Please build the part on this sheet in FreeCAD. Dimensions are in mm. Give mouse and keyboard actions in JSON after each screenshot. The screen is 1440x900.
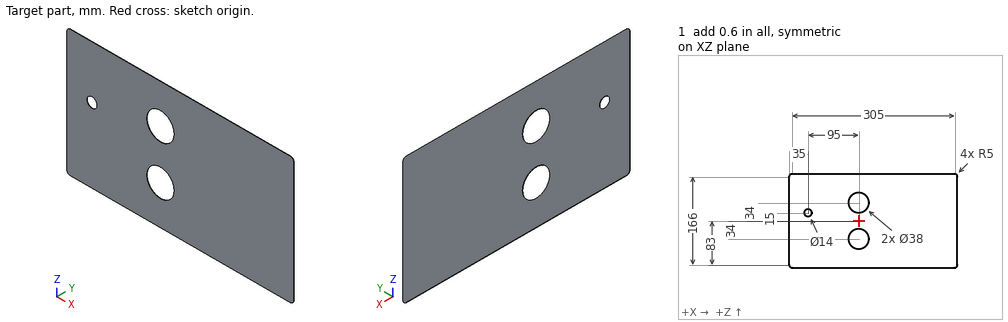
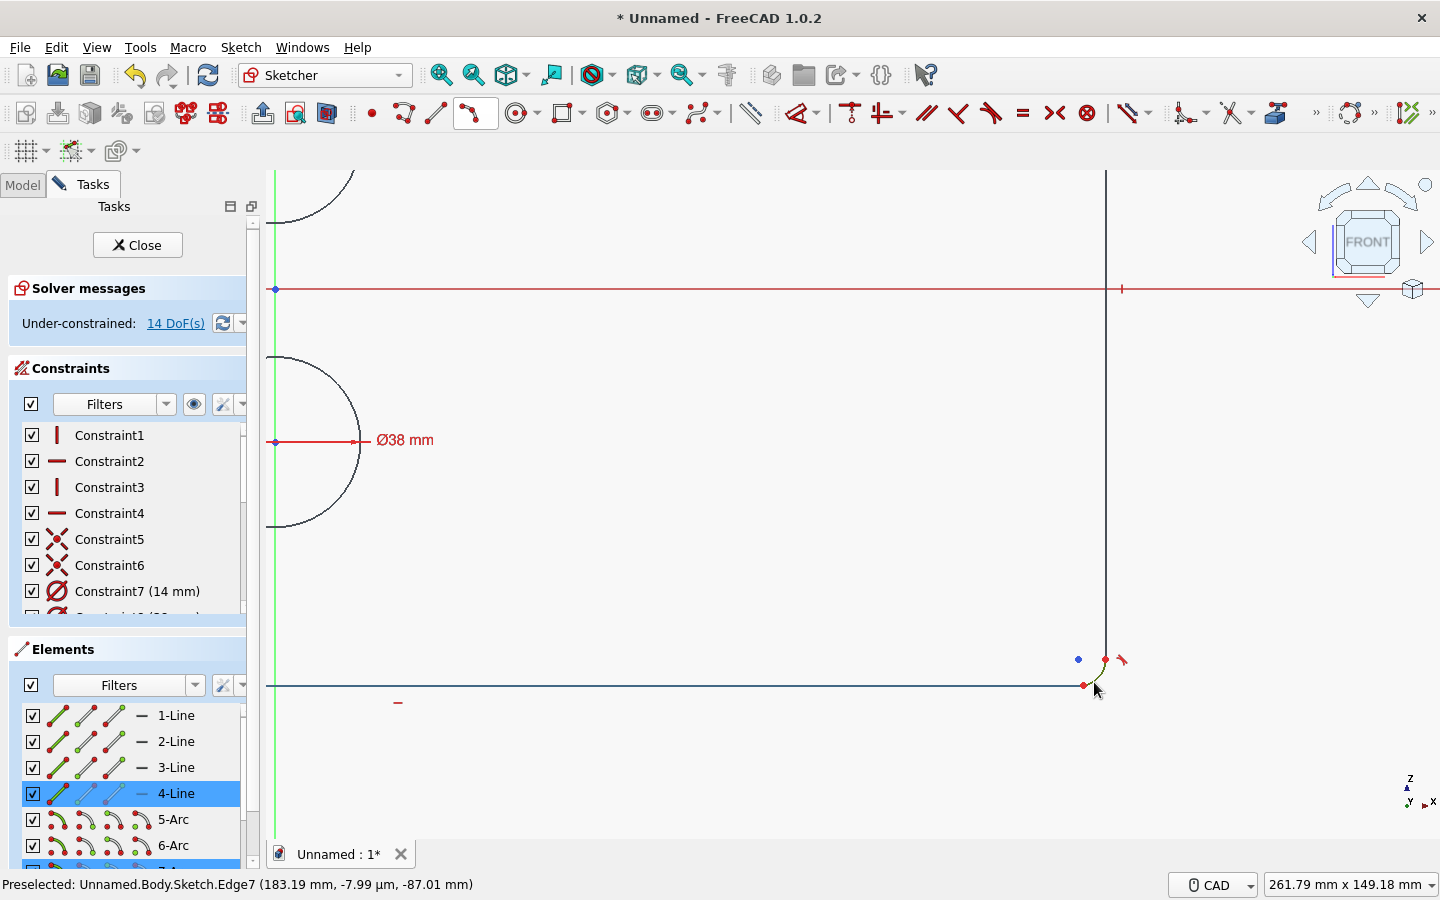
{"action": "left_click", "coordinate": [992, 114]}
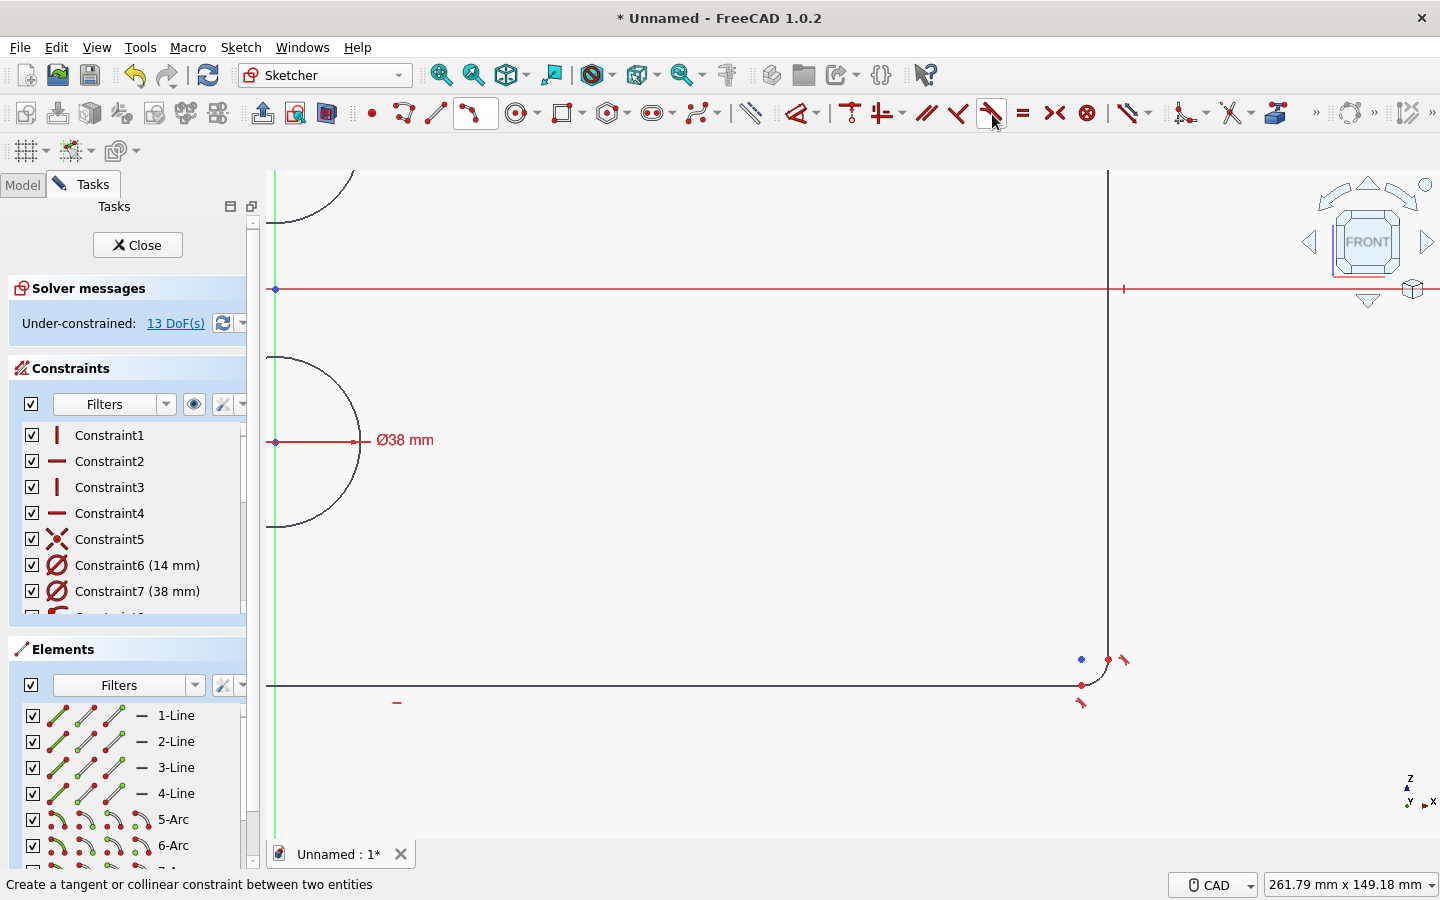
{"action": "left_click", "coordinate": [671, 686]}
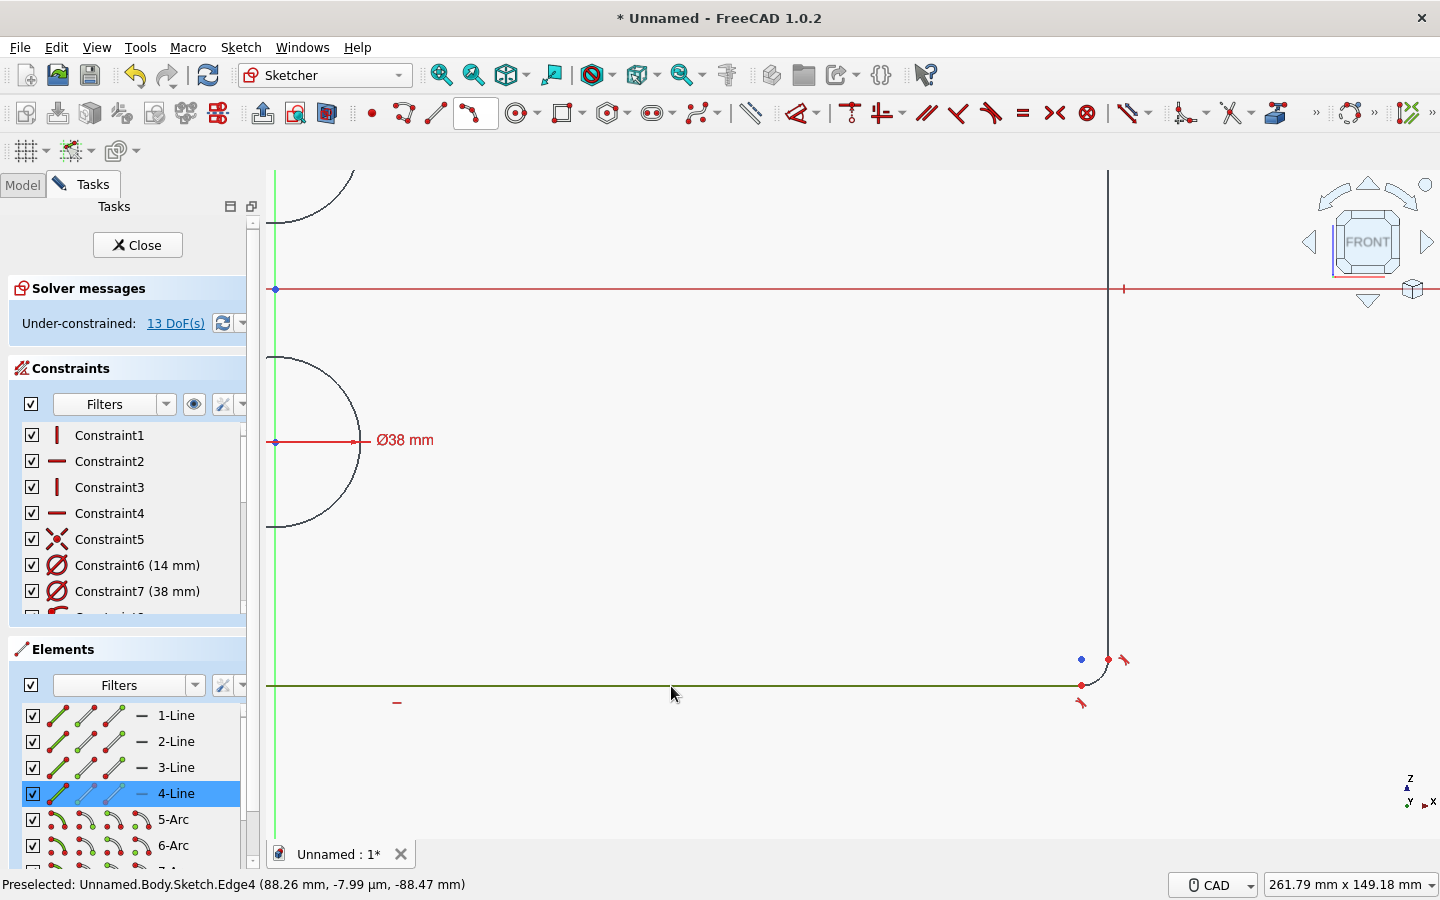
{"action": "scroll", "coordinate": [1099, 680], "scroll_direction": "down", "scroll_amount": 4}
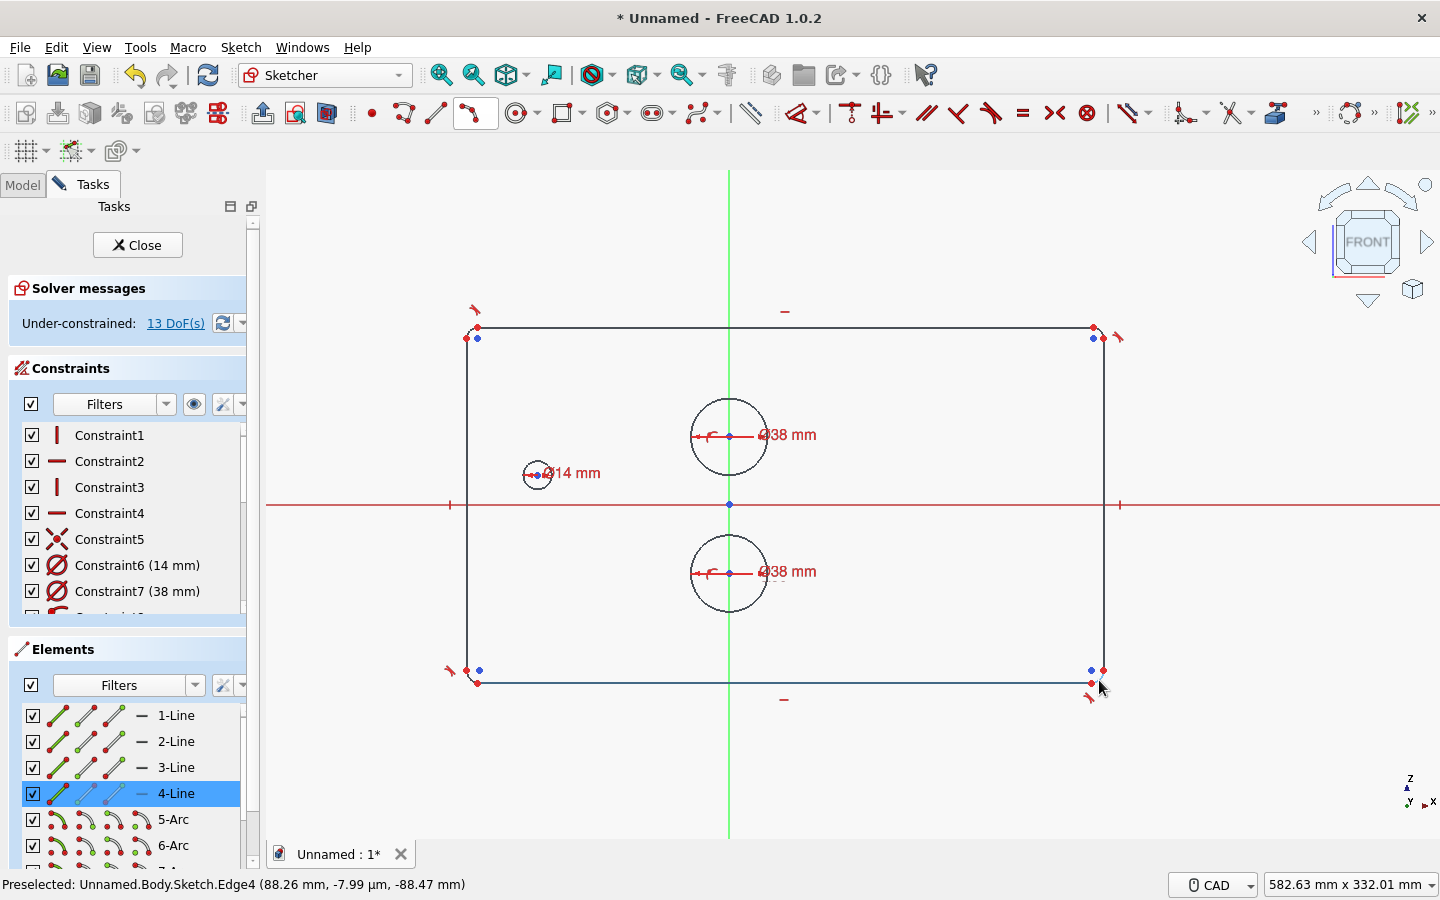
{"action": "scroll", "coordinate": [468, 676], "scroll_direction": "up", "scroll_amount": 5}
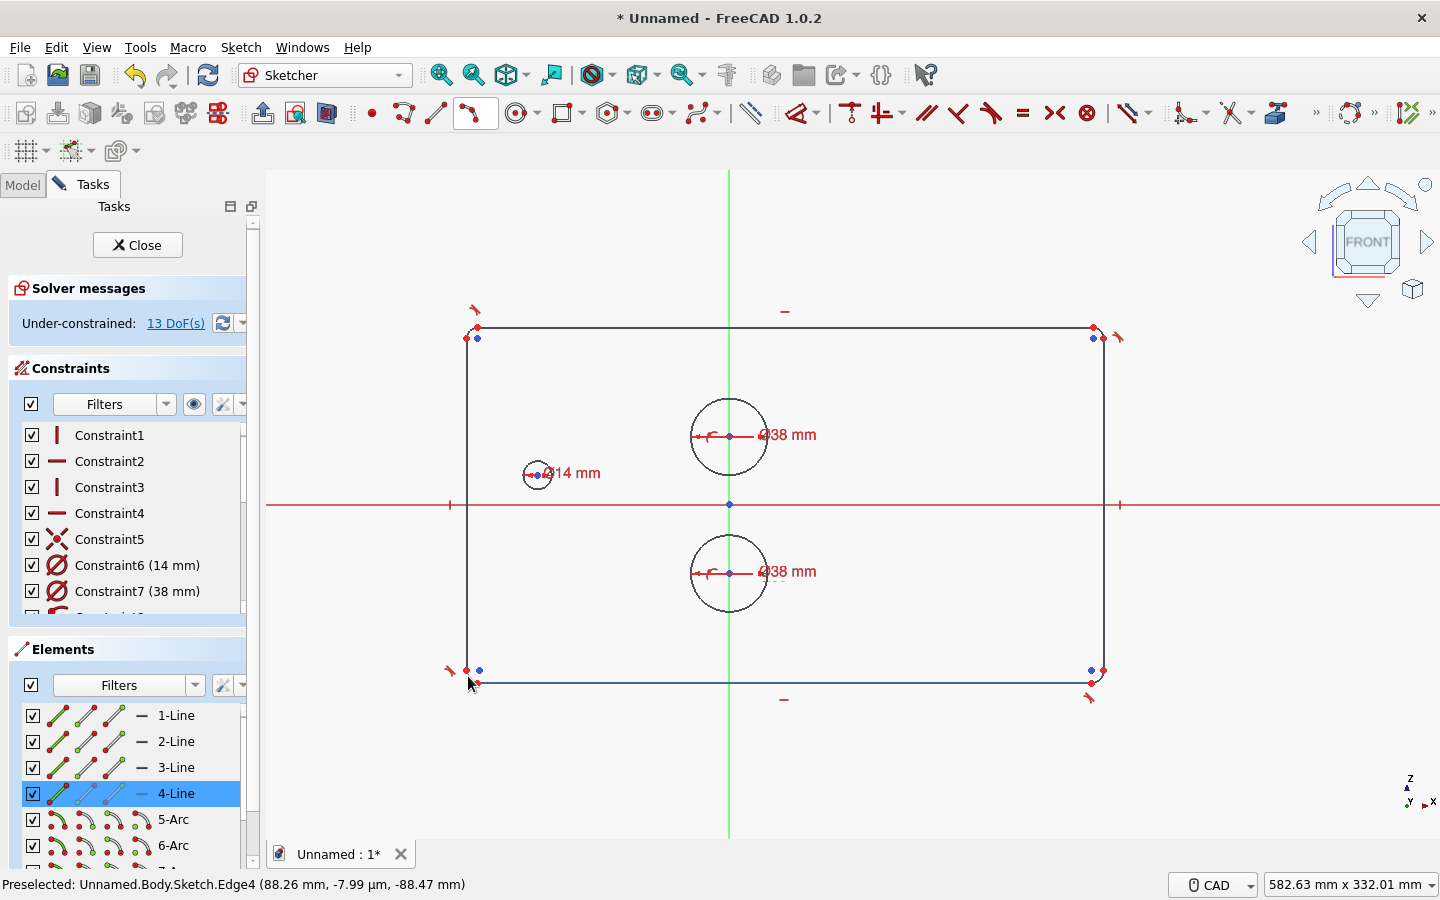
{"action": "left_click", "coordinate": [468, 675]}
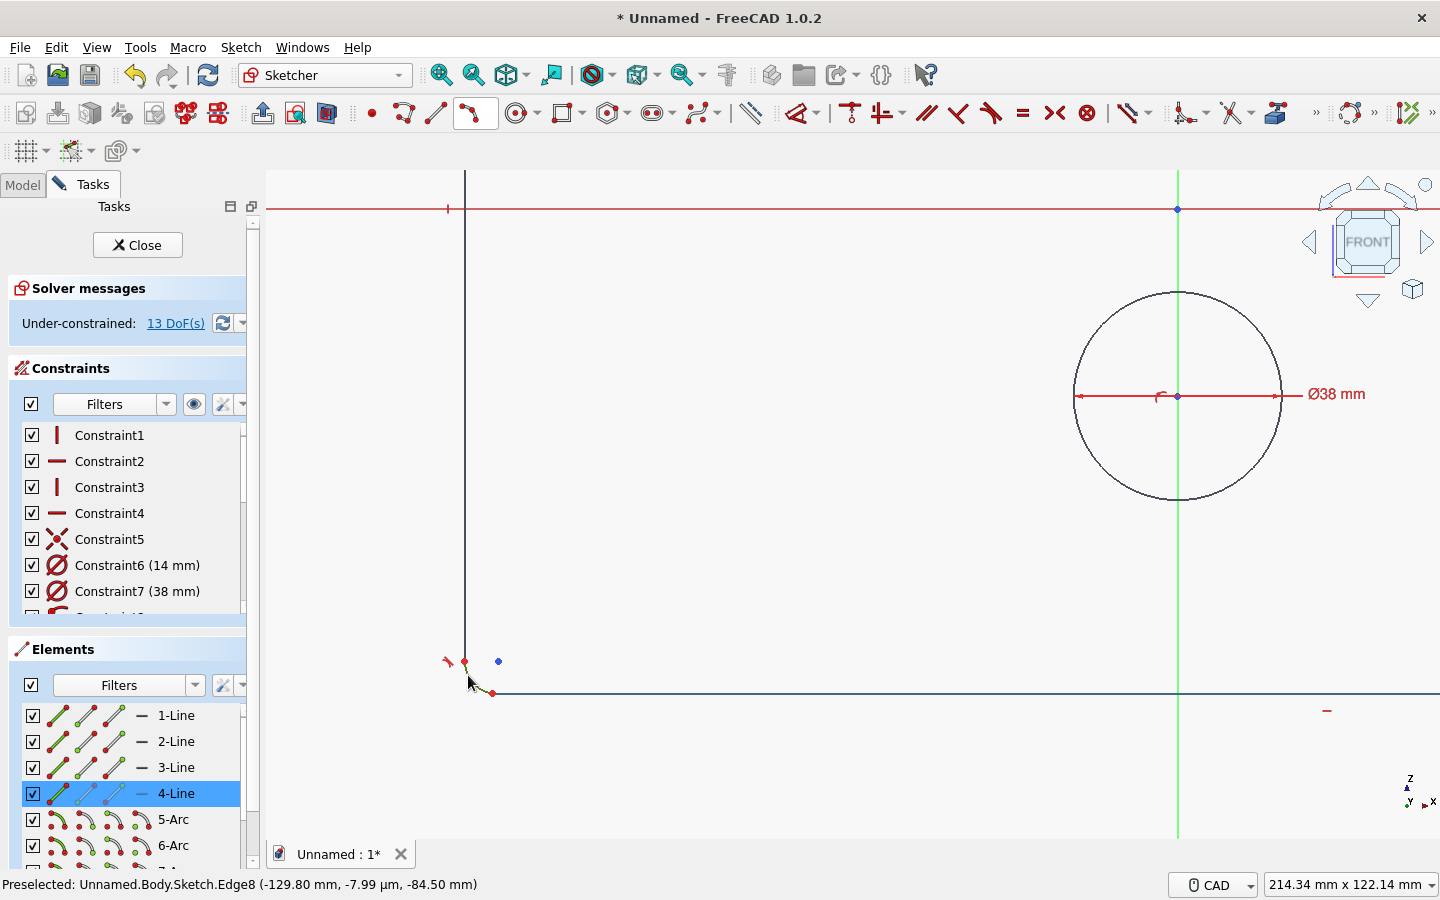
{"action": "left_click", "coordinate": [992, 114]}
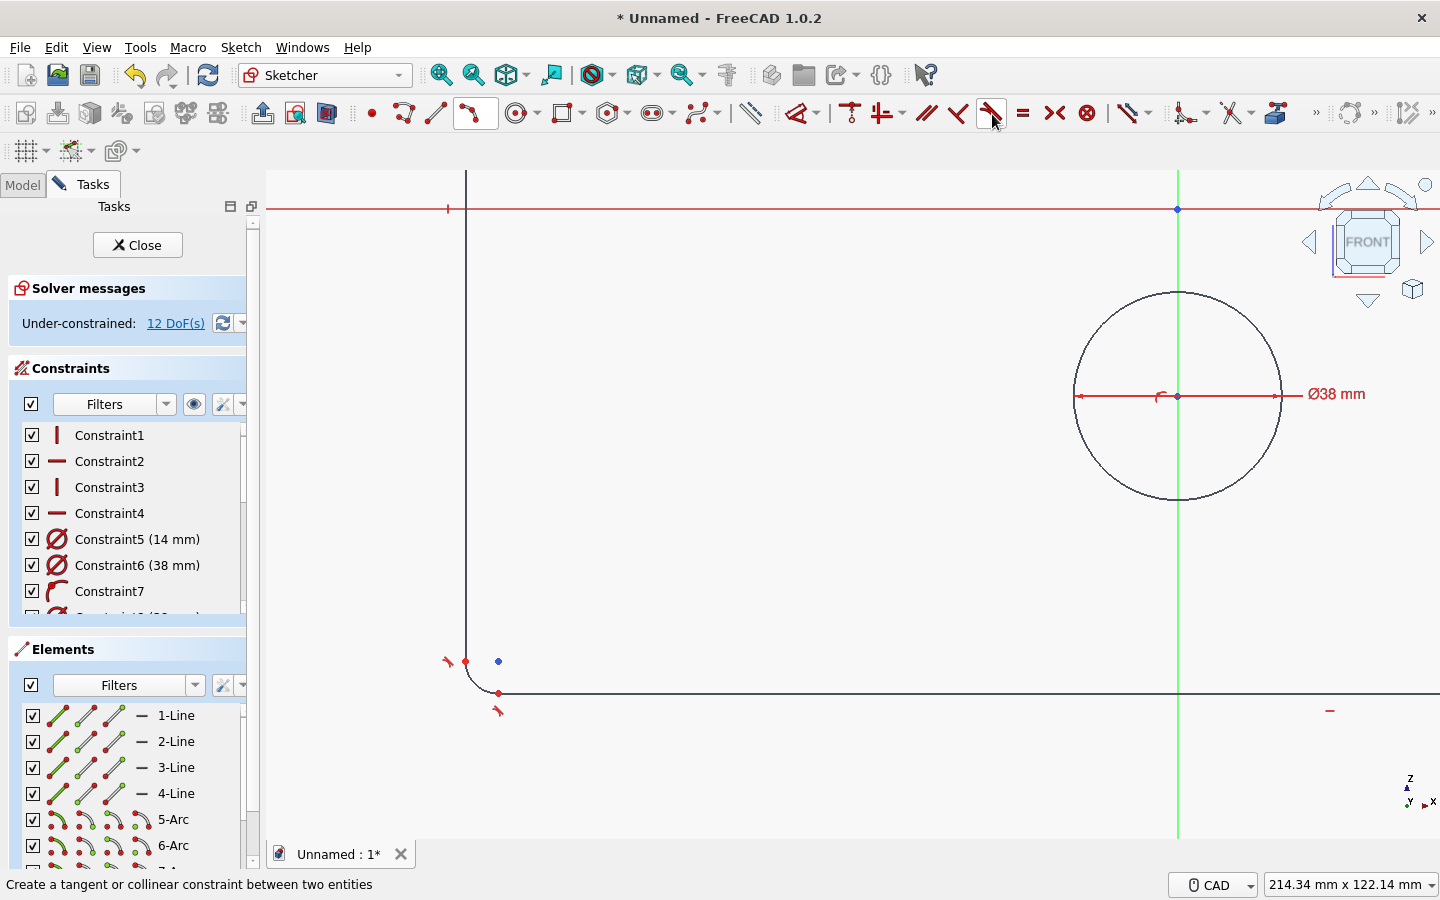
{"action": "scroll", "coordinate": [468, 676], "scroll_direction": "down", "scroll_amount": 5}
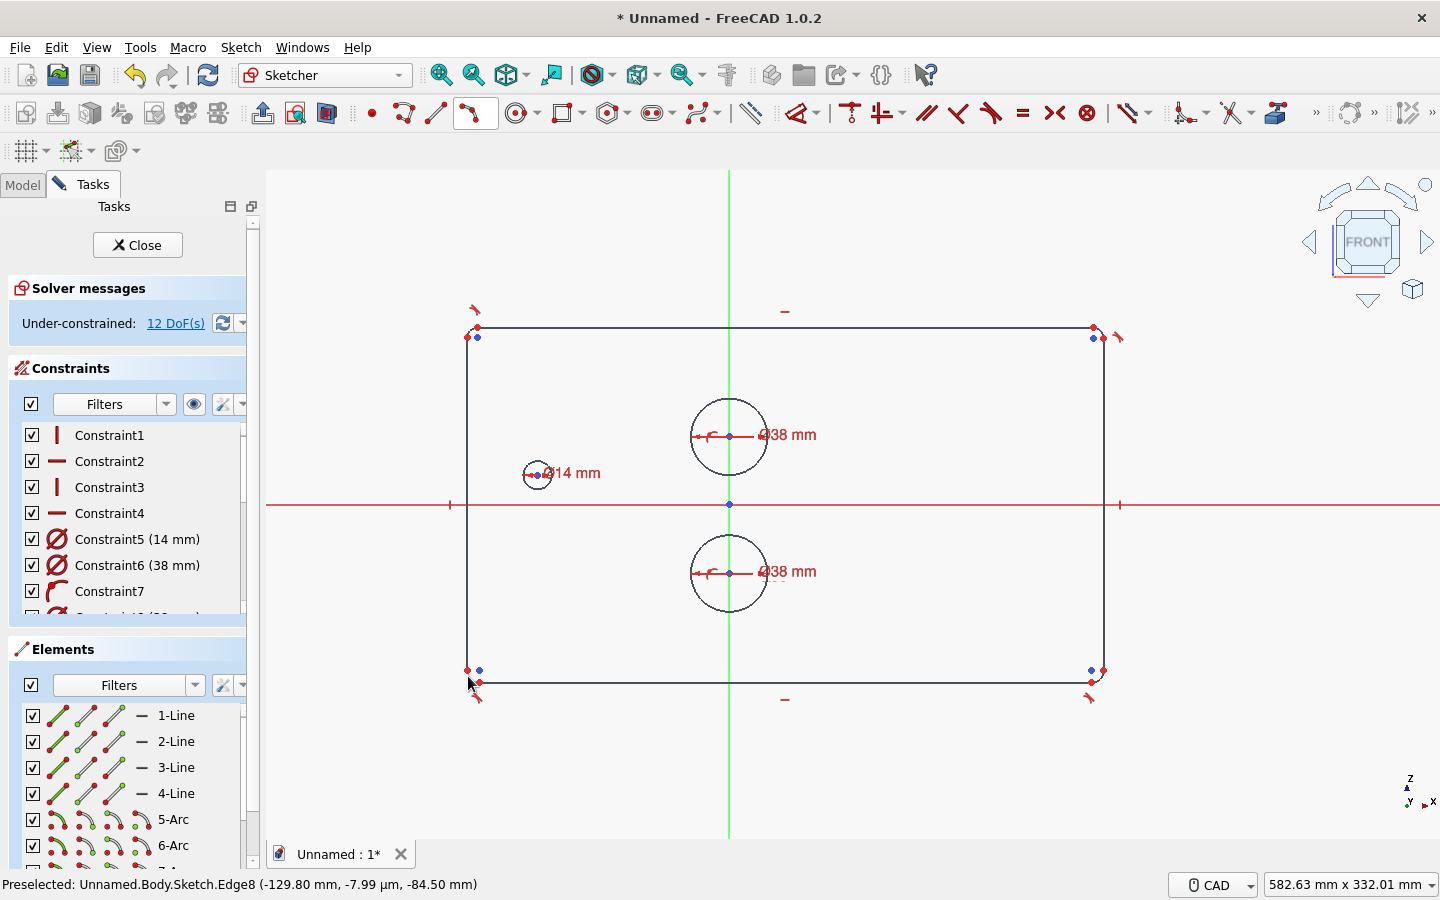
{"action": "scroll", "coordinate": [473, 329], "scroll_direction": "up", "scroll_amount": 6}